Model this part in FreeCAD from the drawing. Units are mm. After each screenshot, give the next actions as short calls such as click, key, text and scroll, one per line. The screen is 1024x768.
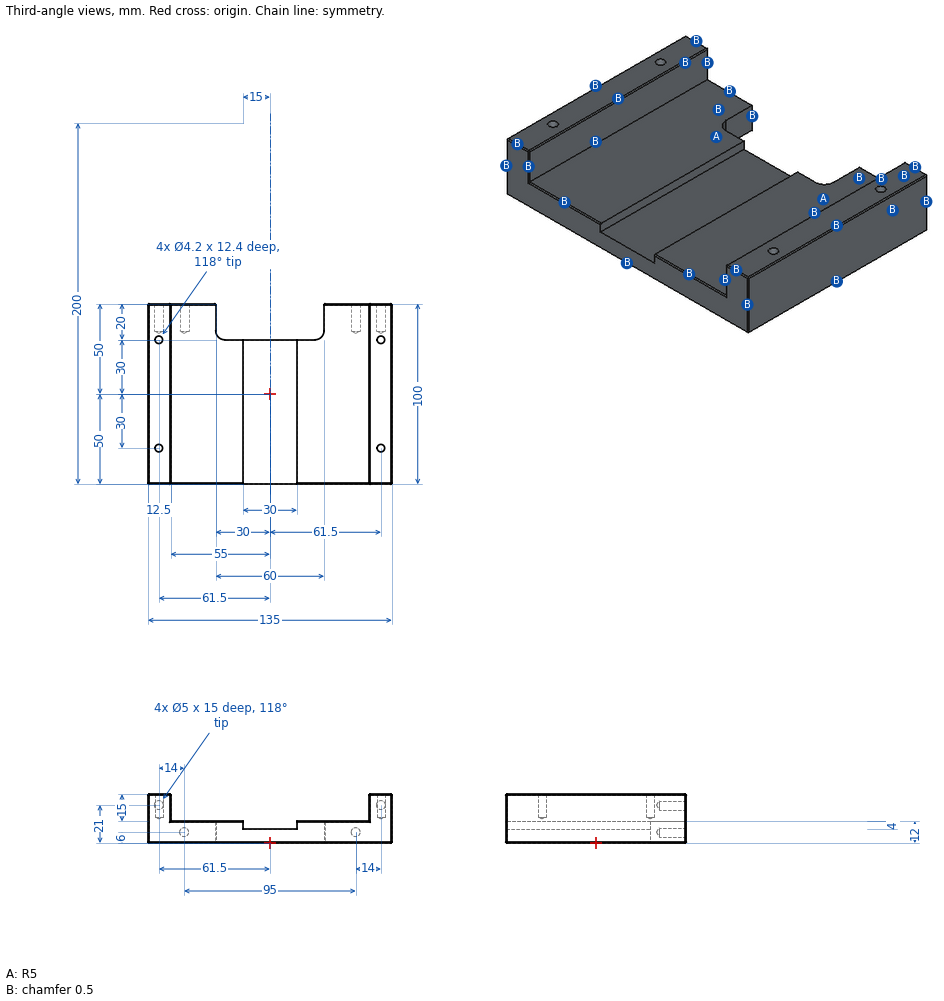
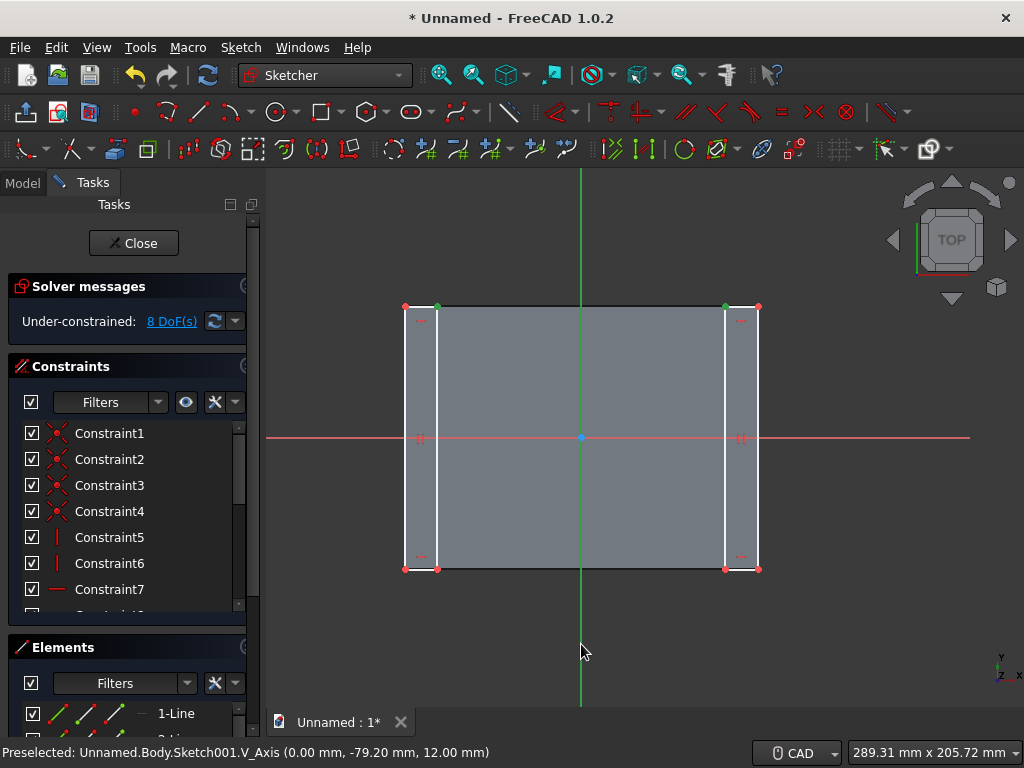
key(s)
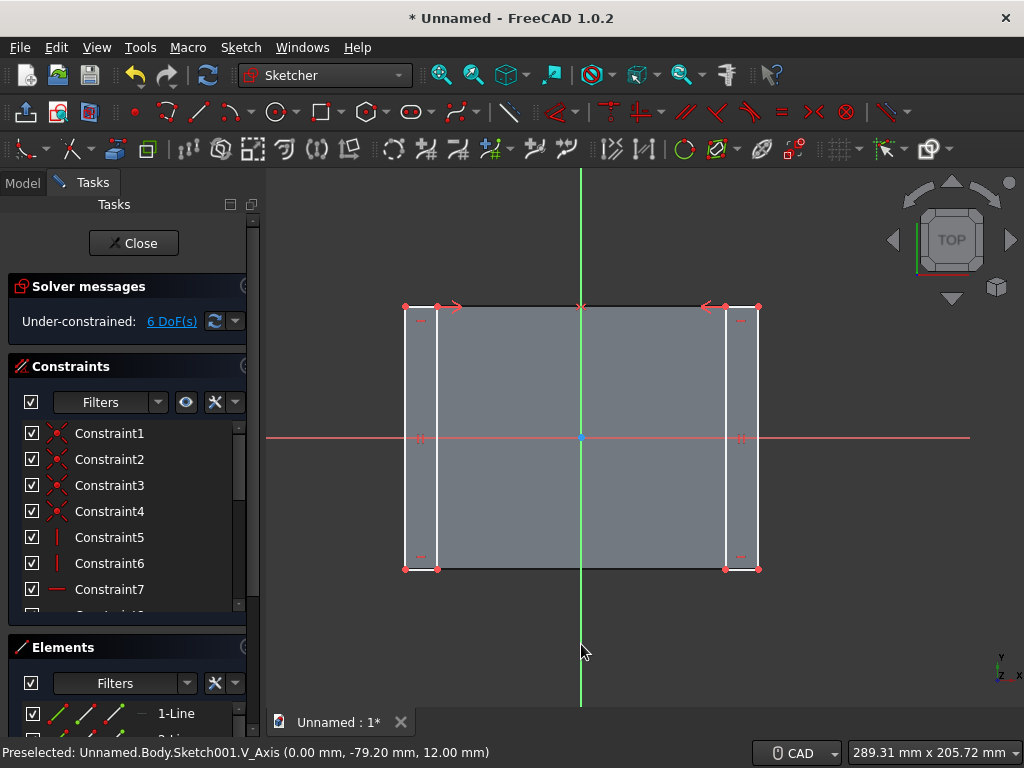
click(405, 570)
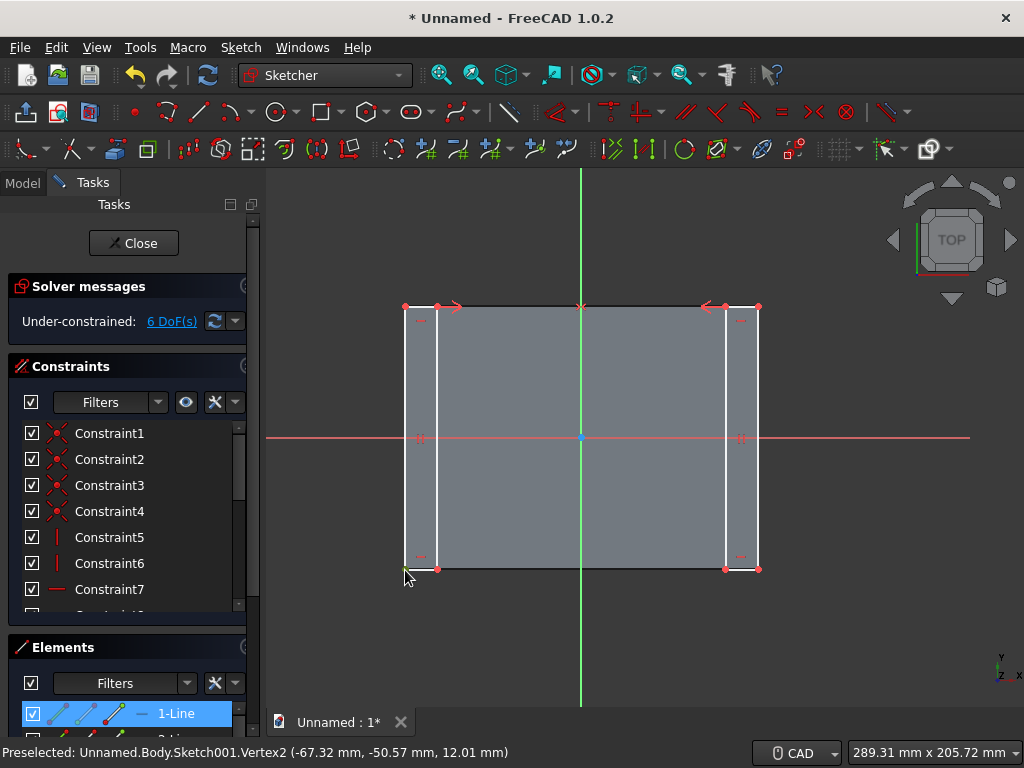
click(758, 570)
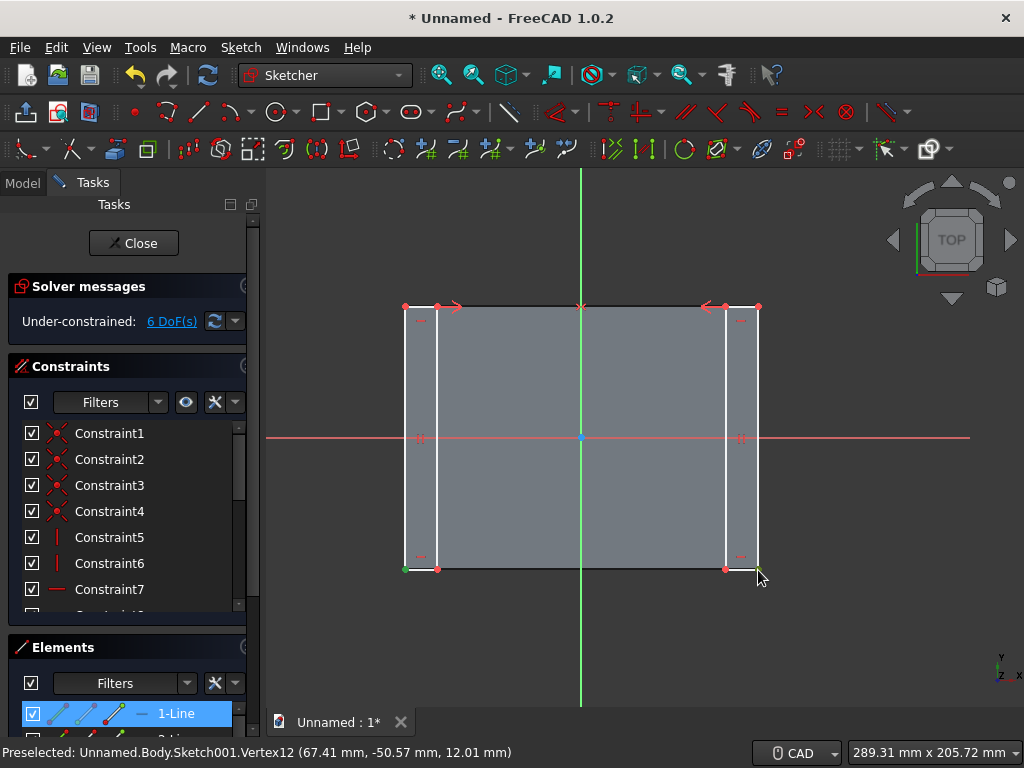
click(581, 644)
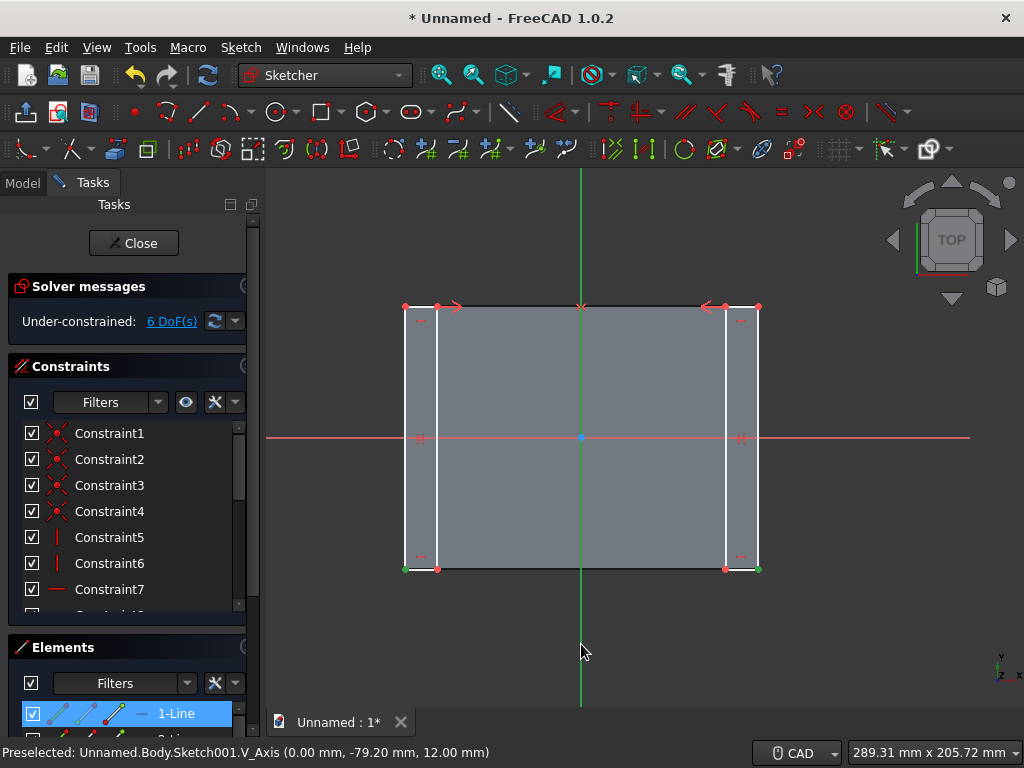
click(814, 112)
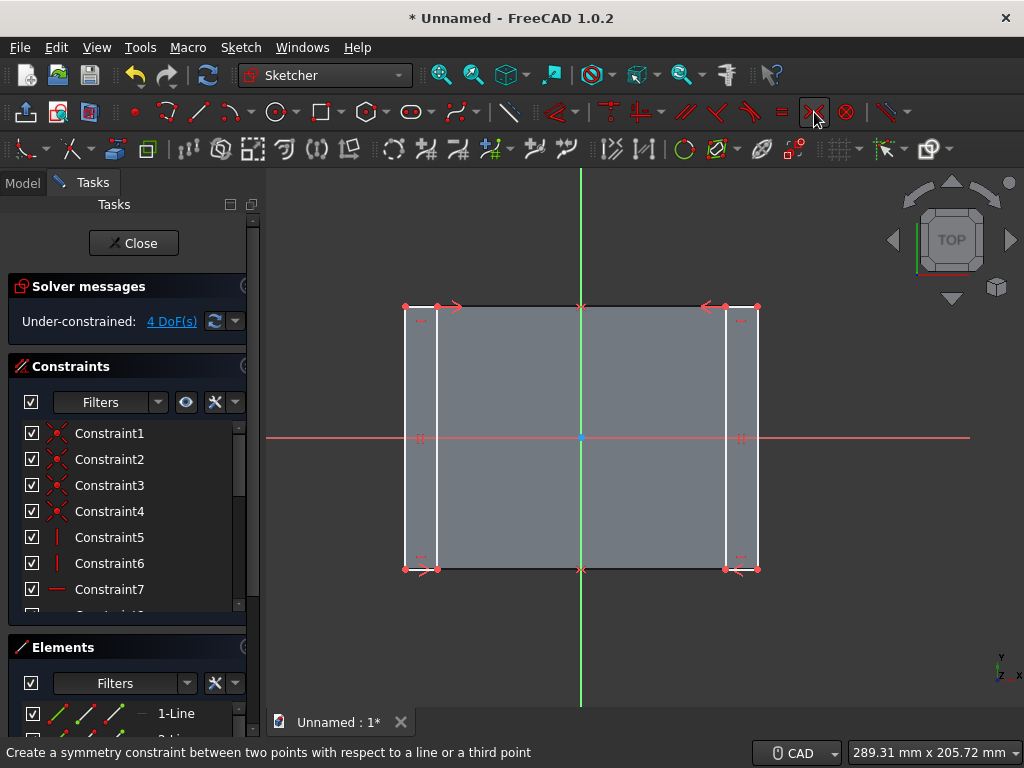
key(d)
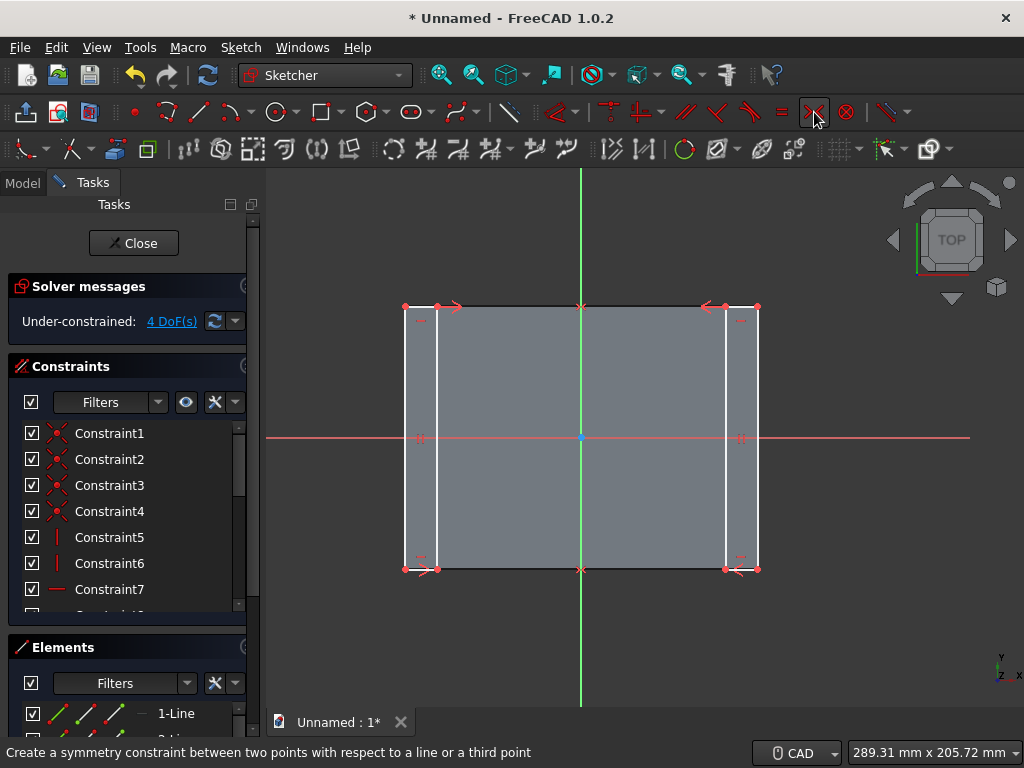
click(405, 386)
click(371, 378)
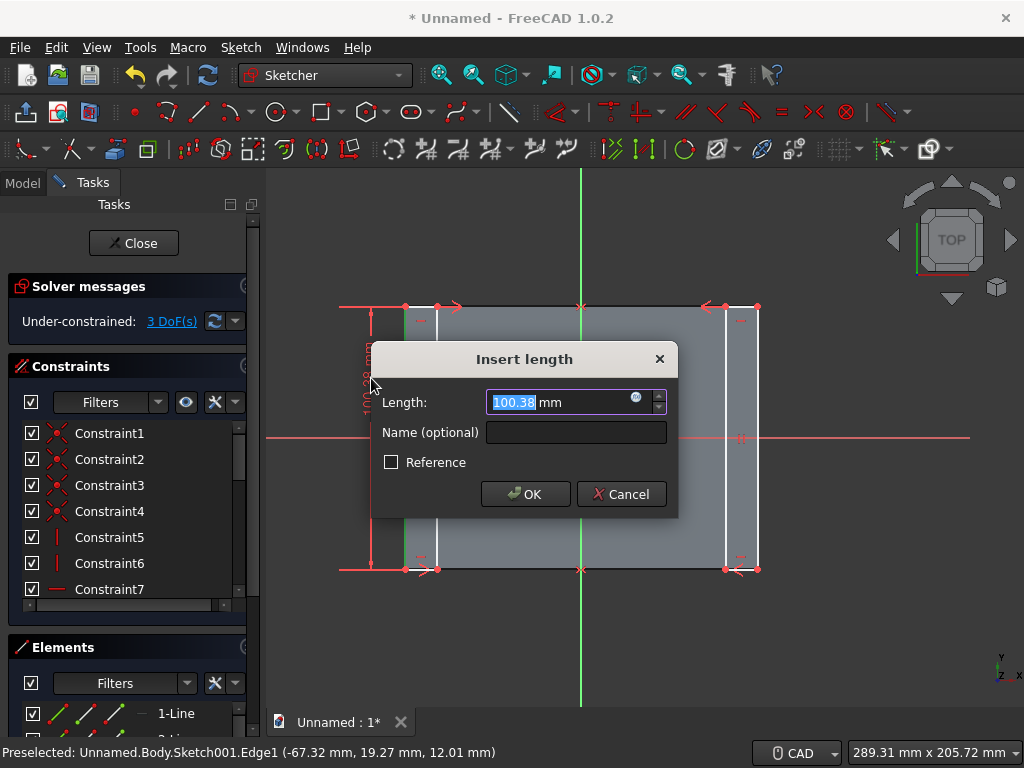
text(100)
key(Return)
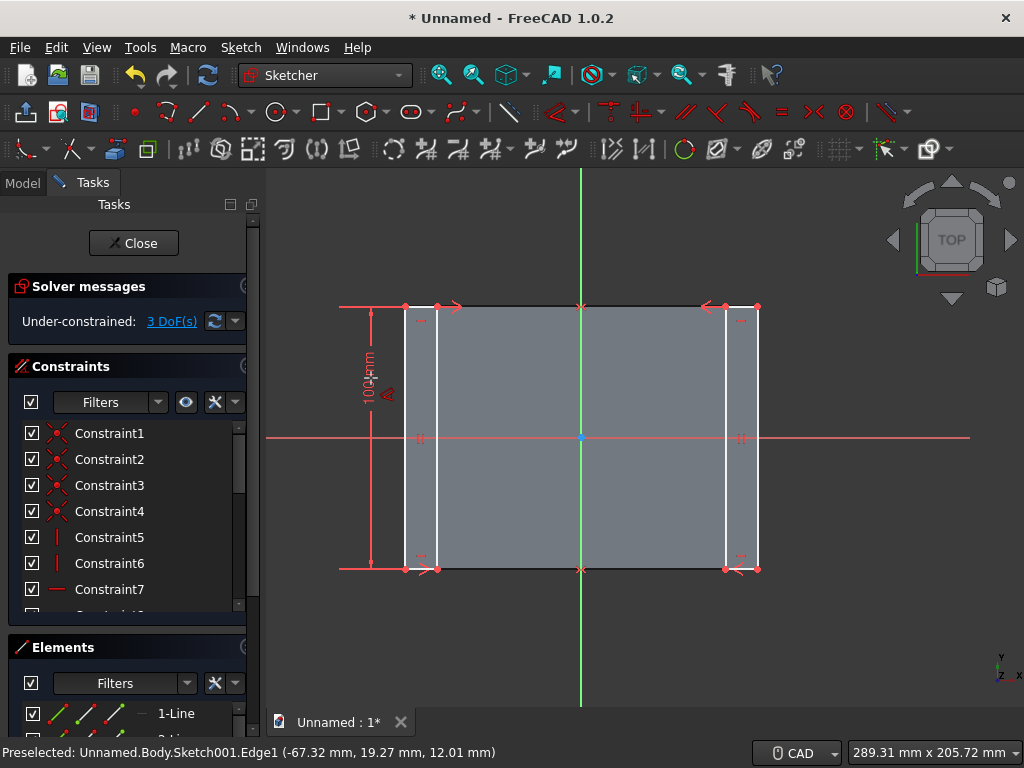
click(405, 307)
click(371, 342)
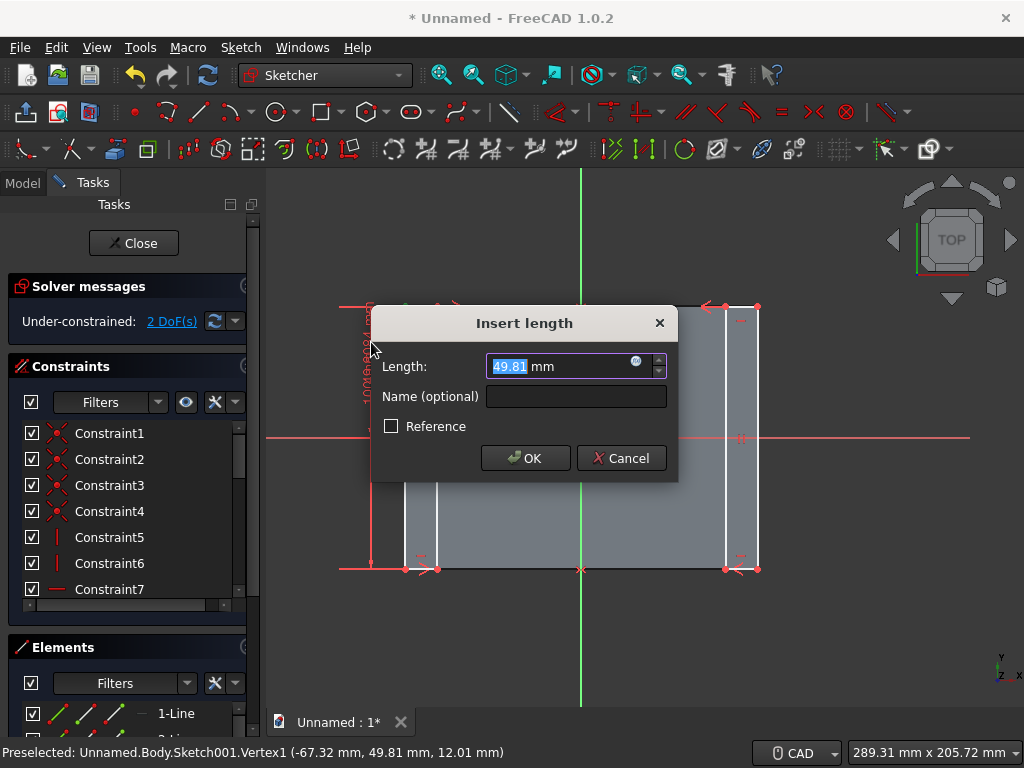
text(50)
key(Return)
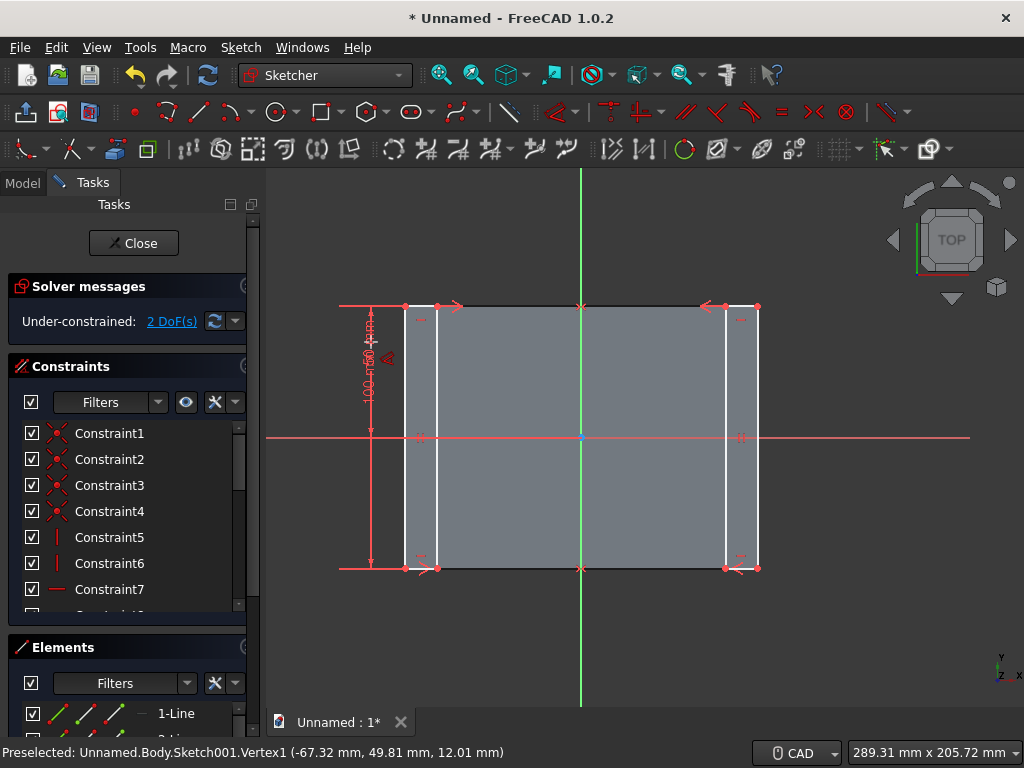
click(437, 569)
click(509, 603)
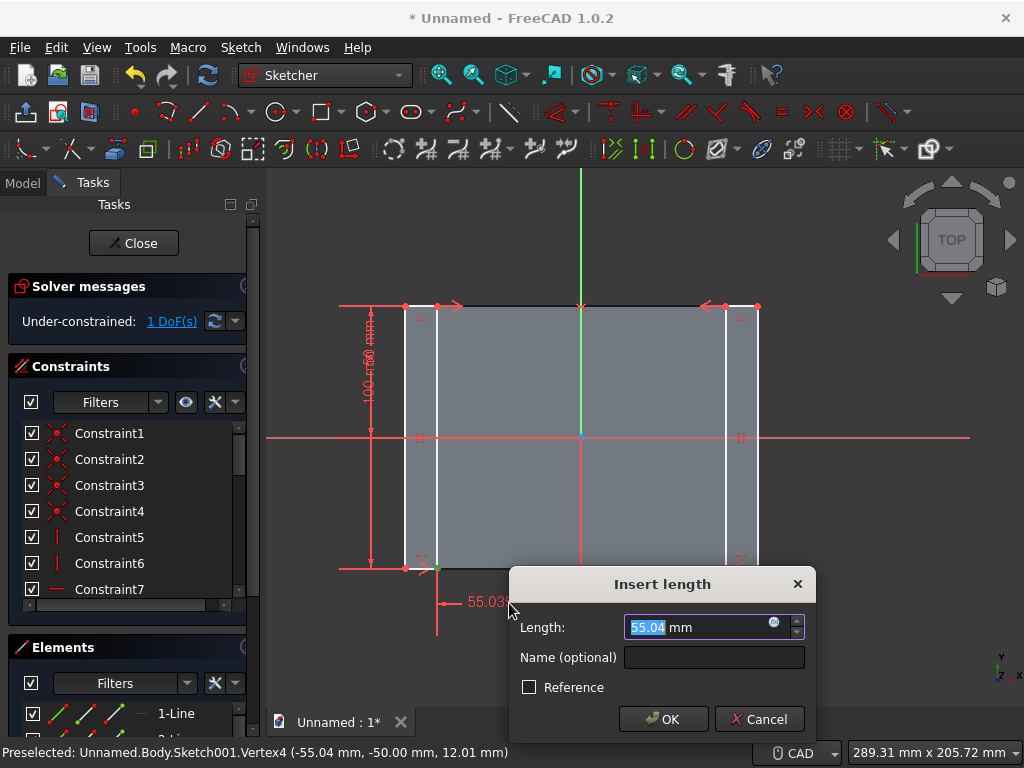
text(55)
key(Return)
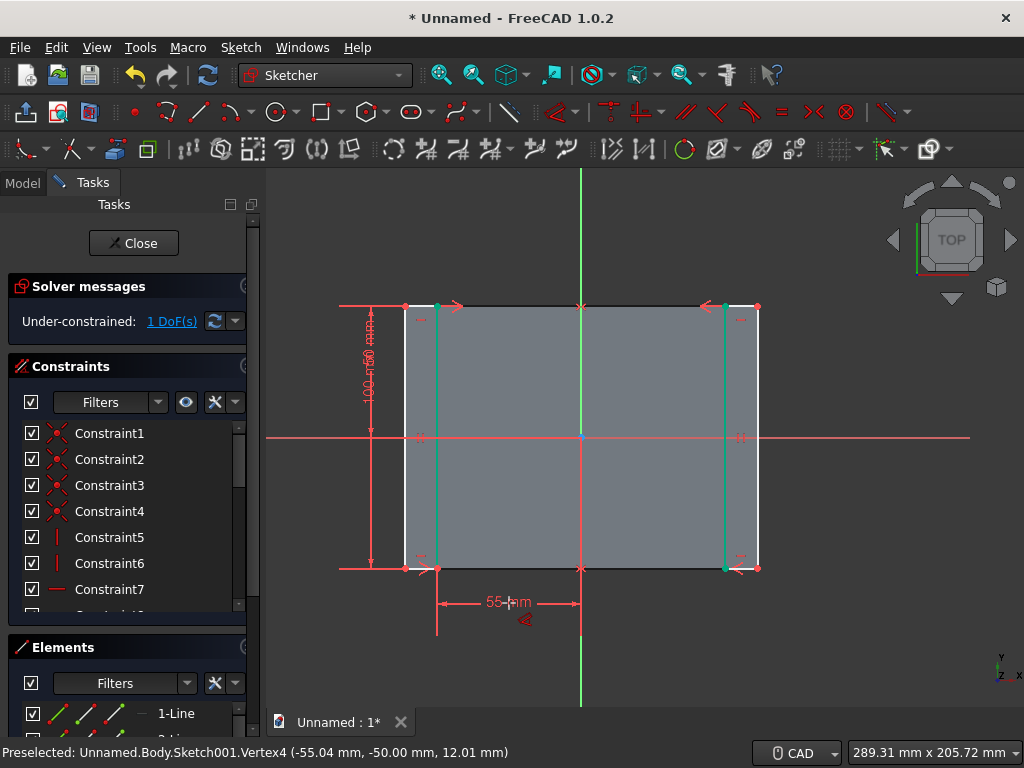
scroll(415, 569, up, 2)